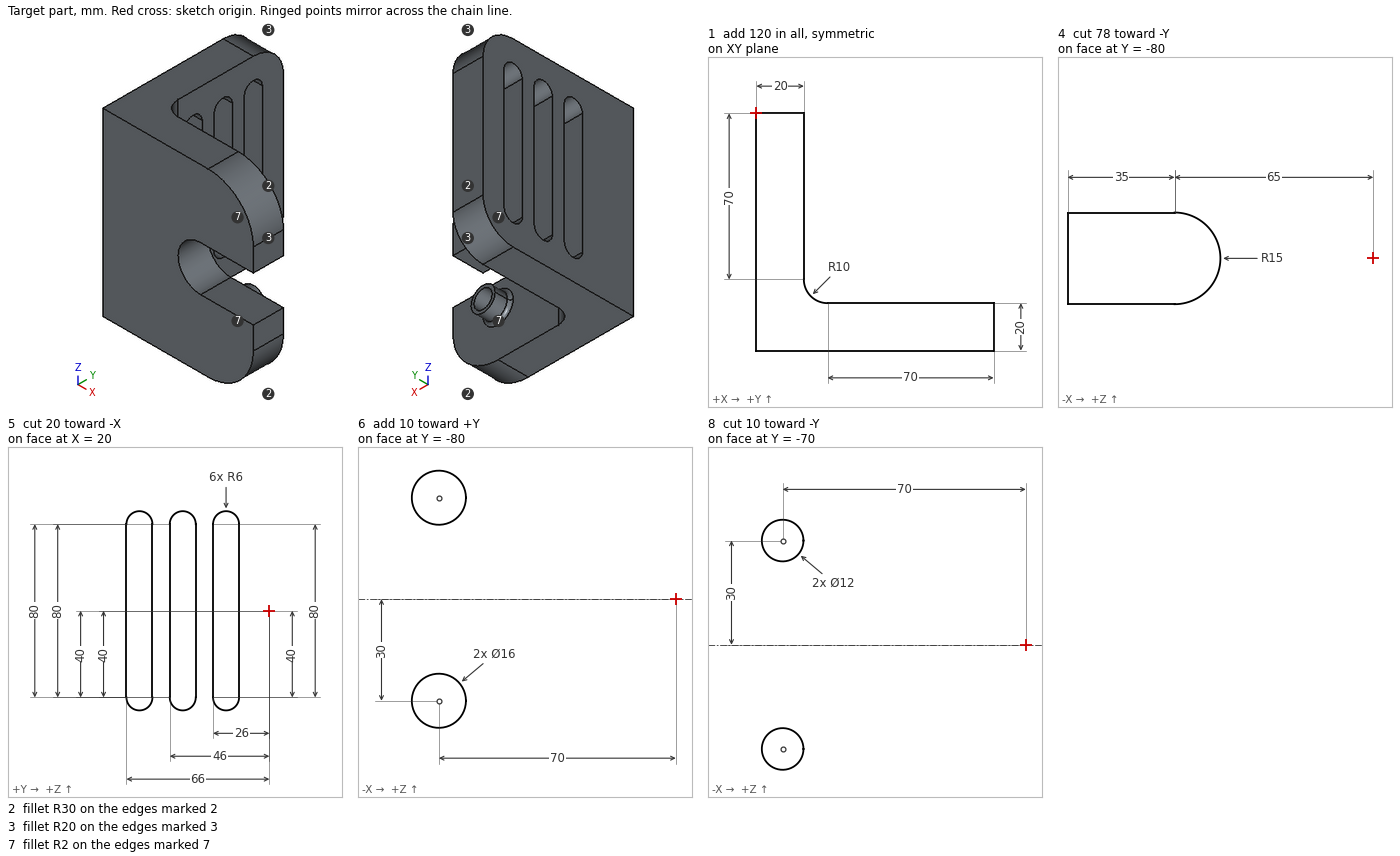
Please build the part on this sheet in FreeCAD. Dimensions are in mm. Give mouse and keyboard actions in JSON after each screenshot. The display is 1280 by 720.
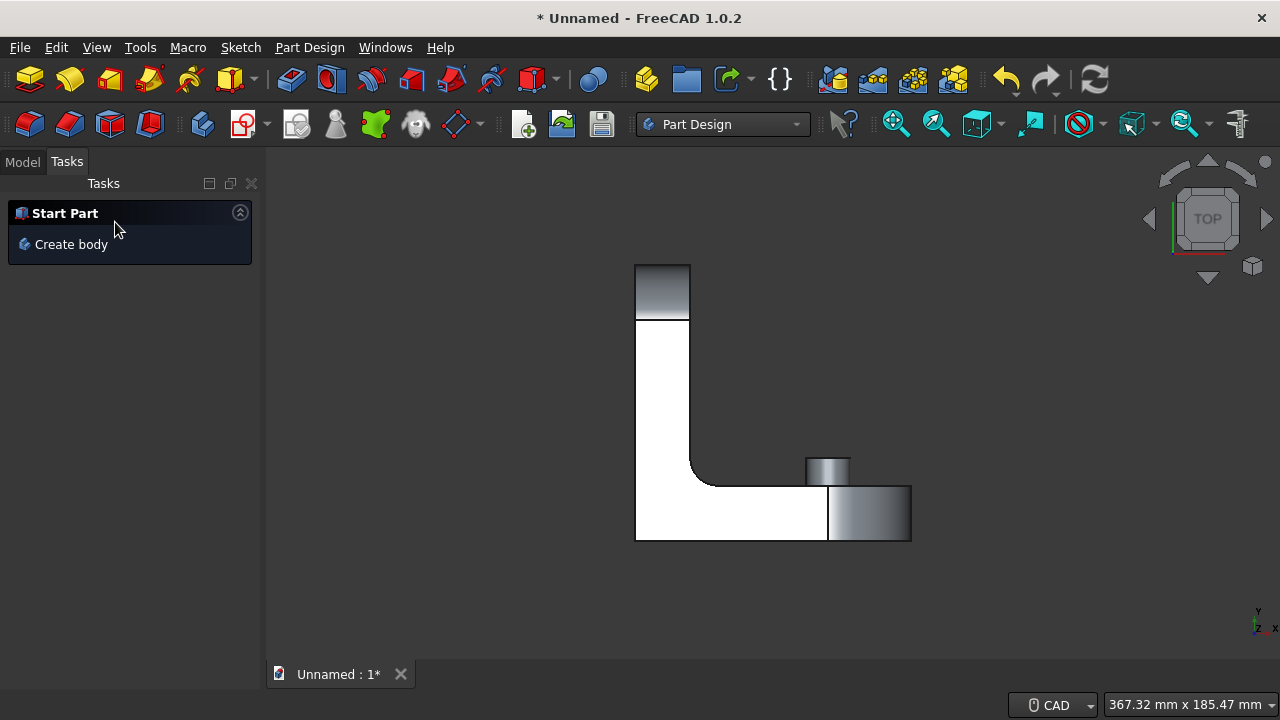
{"action": "key", "text": "1"}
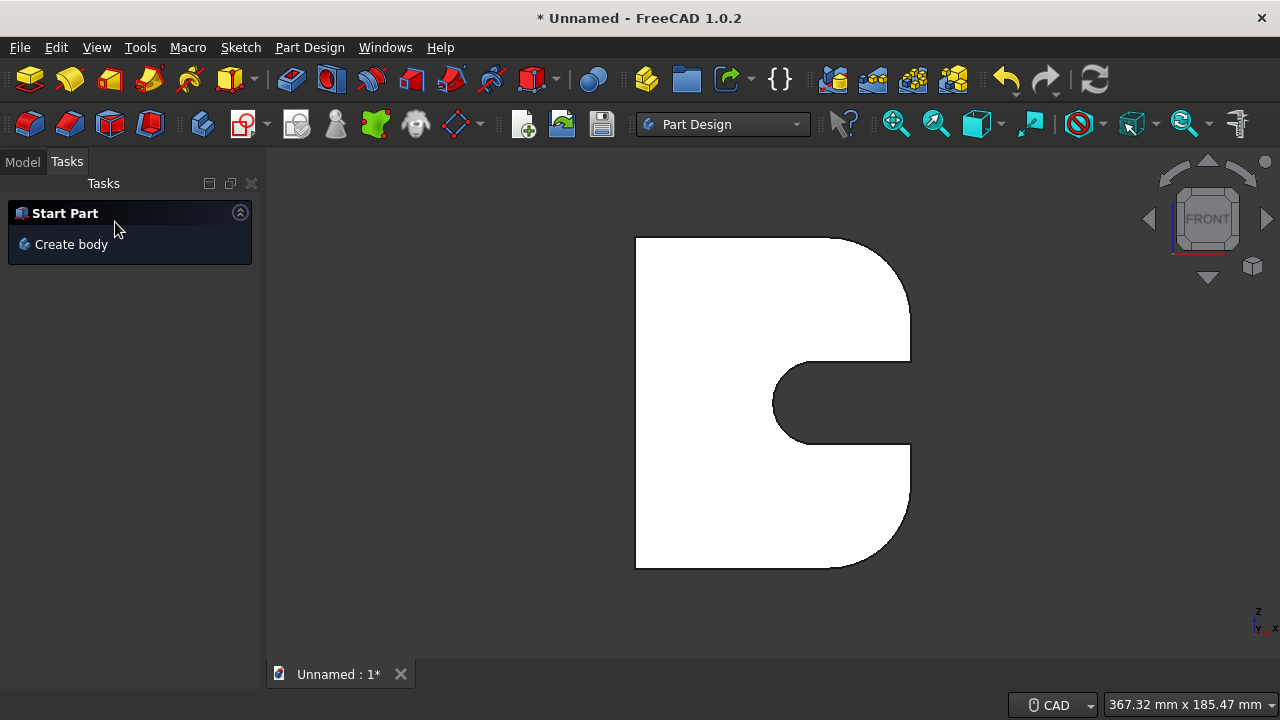
{"action": "key", "text": "3"}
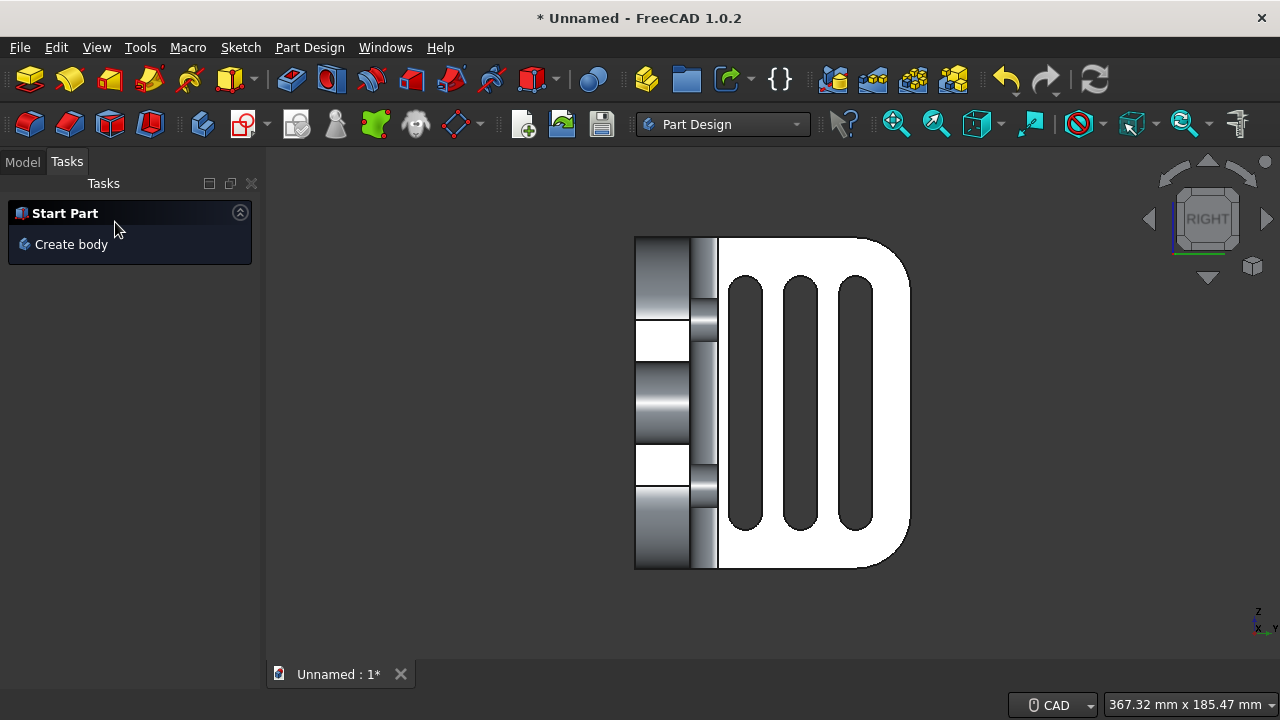
{"action": "key", "text": "5"}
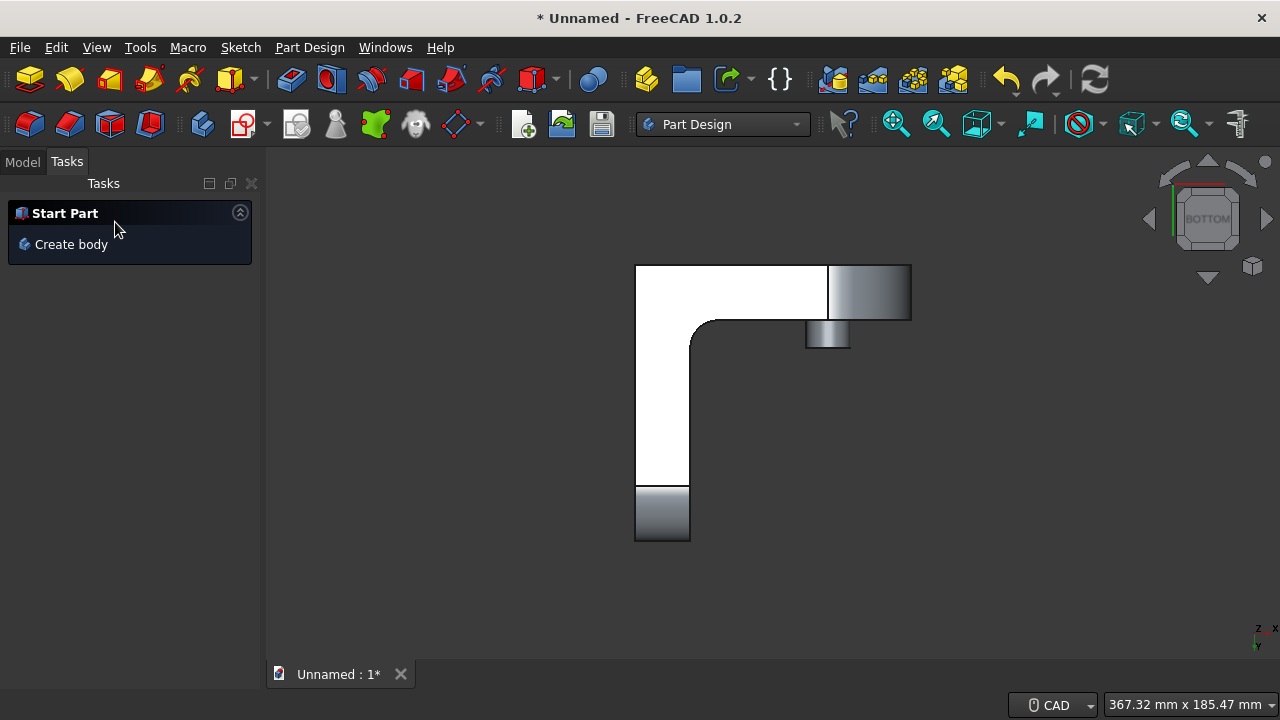
{"action": "key", "text": "4"}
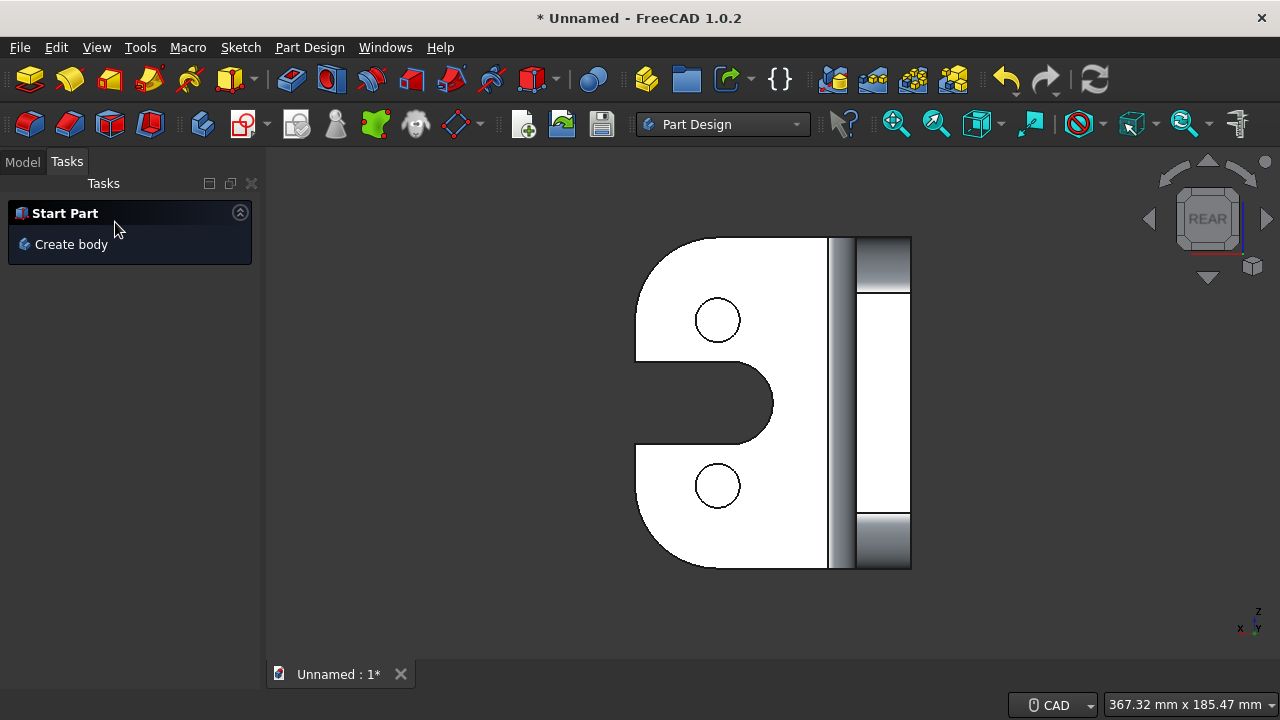
{"action": "key", "text": "6"}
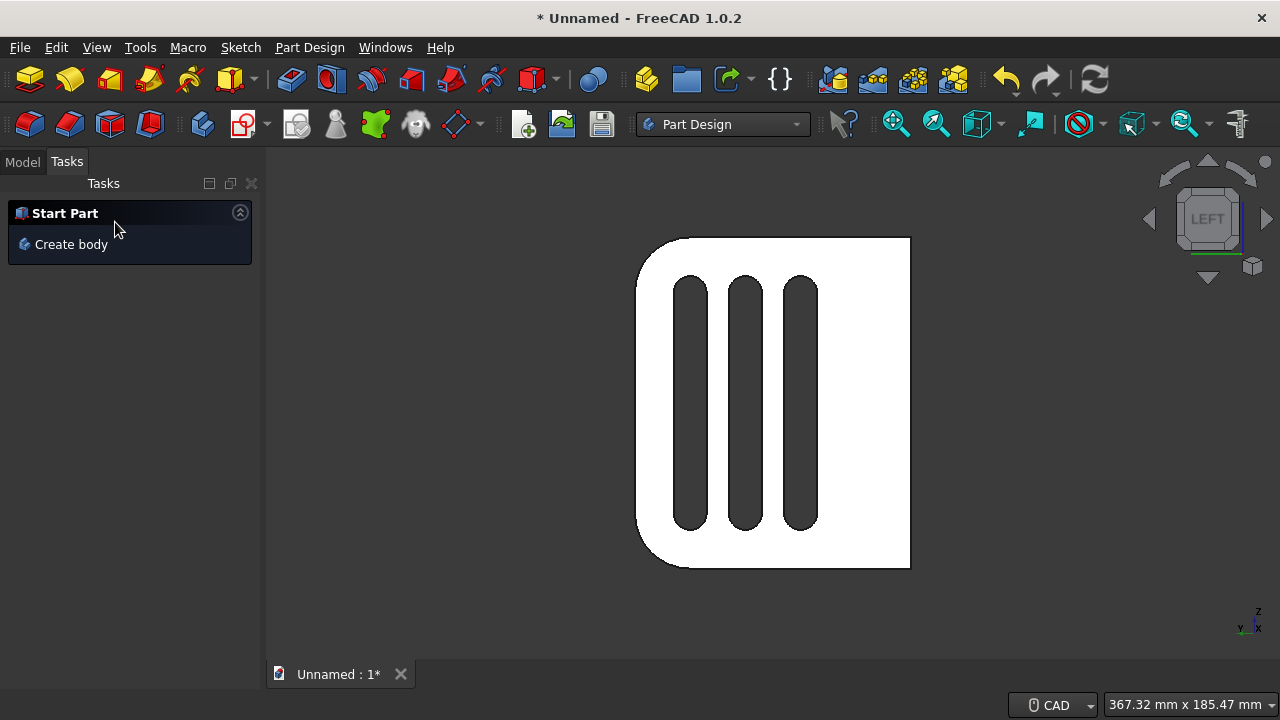
{"action": "key", "text": "v 3"}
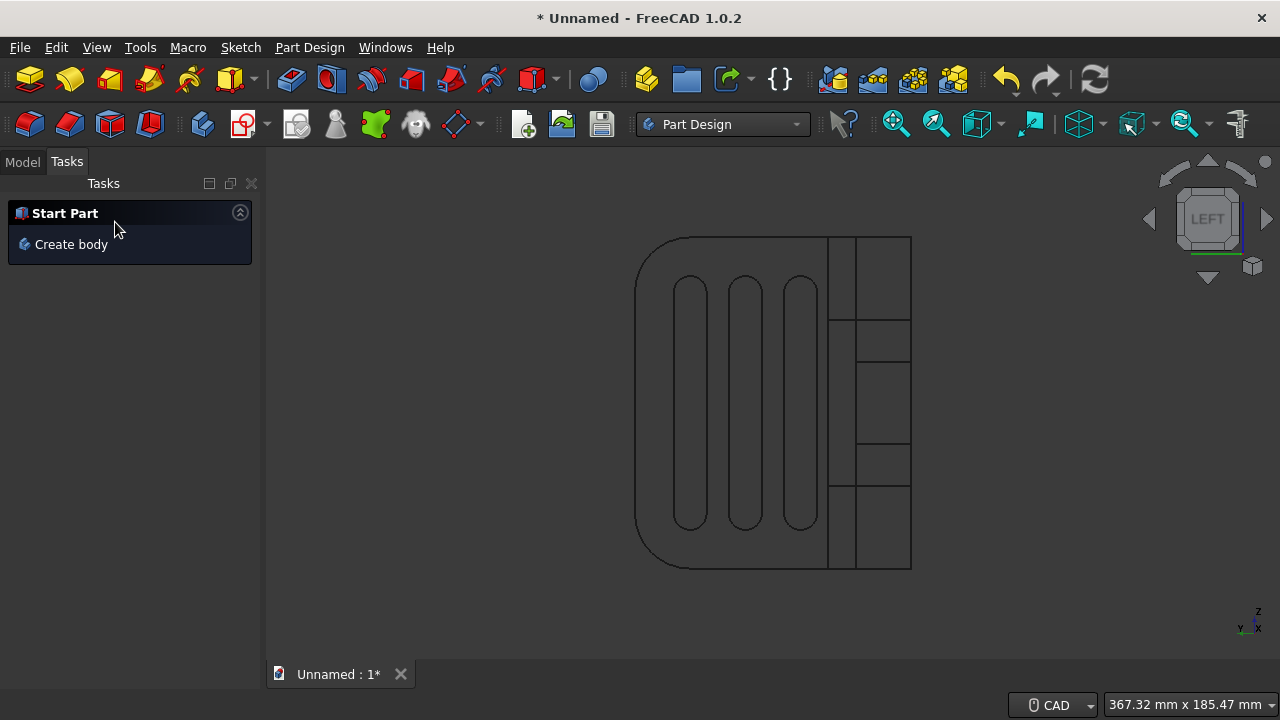
{"action": "key", "text": "0"}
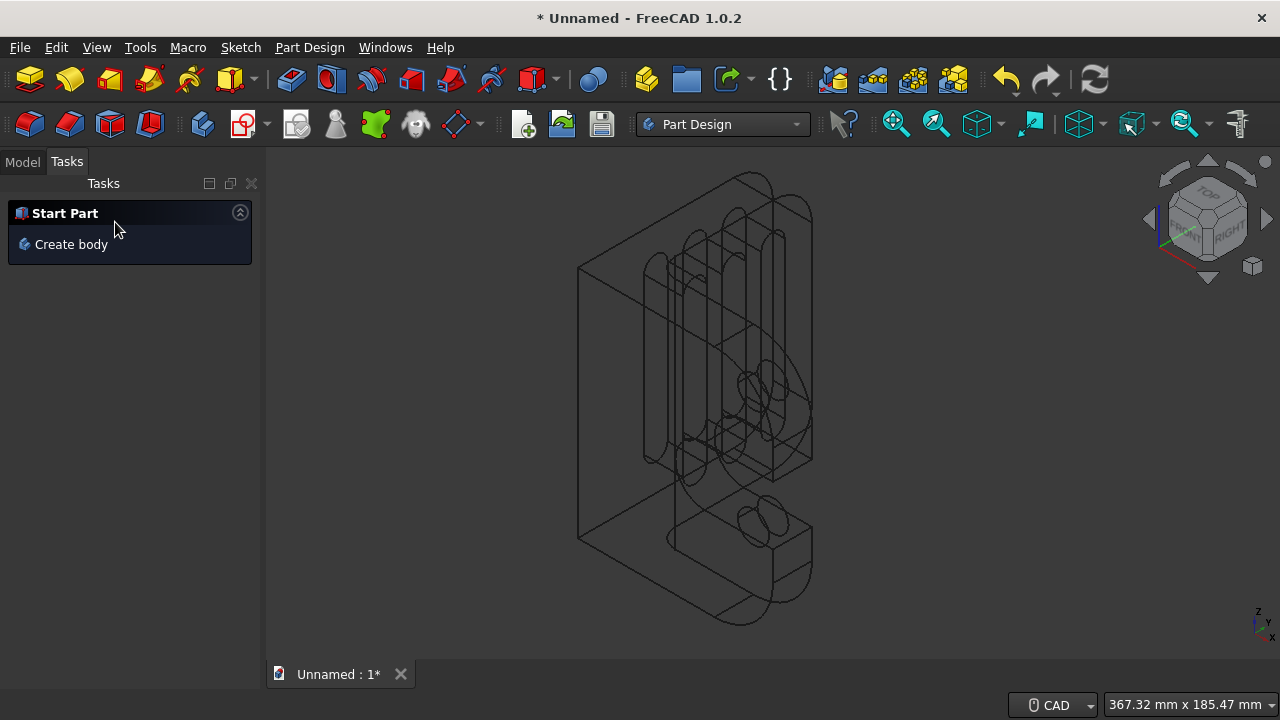
{"action": "left_click", "coordinate": [769, 535]}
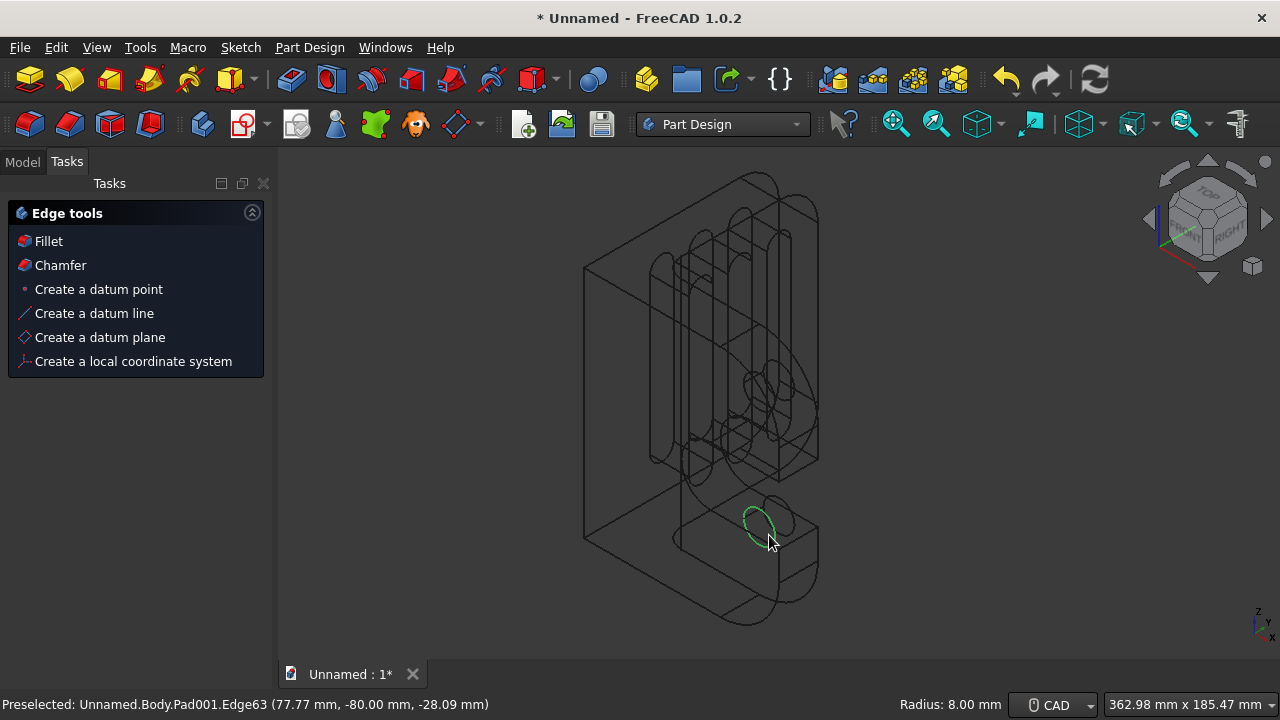
{"action": "left_click", "coordinate": [775, 400], "text": "ctrl"}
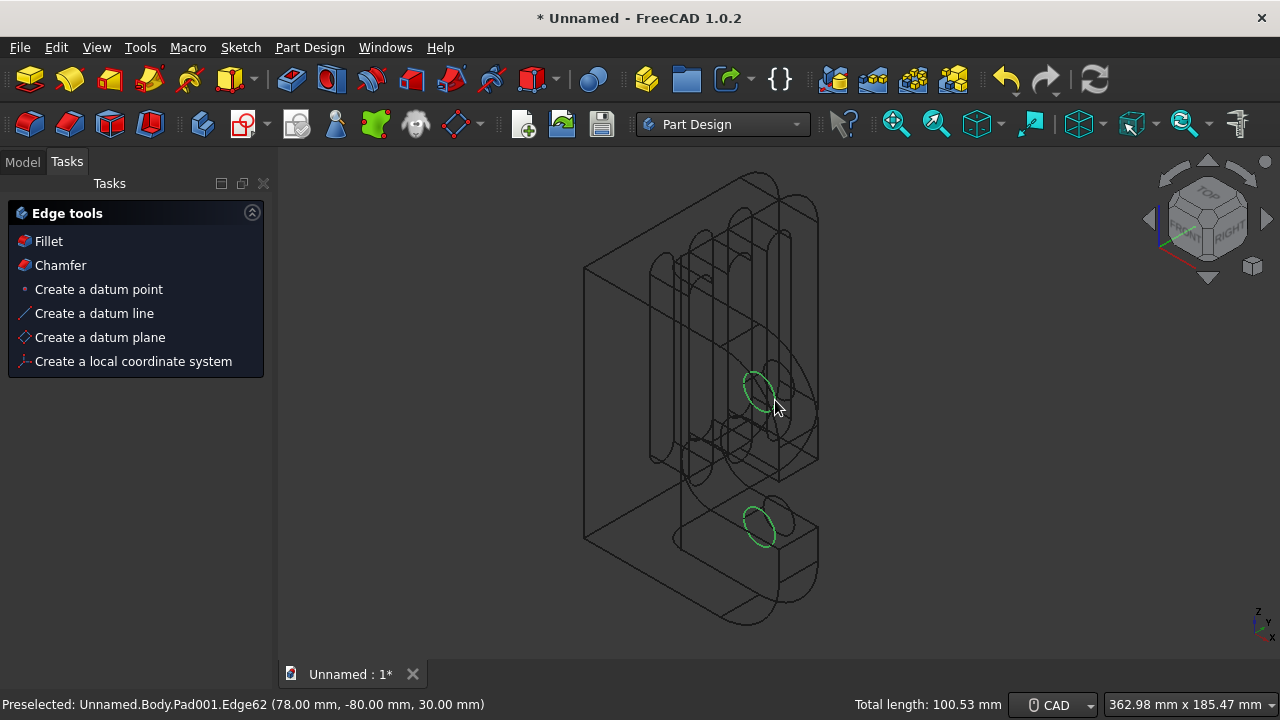
{"action": "key", "text": "v 1"}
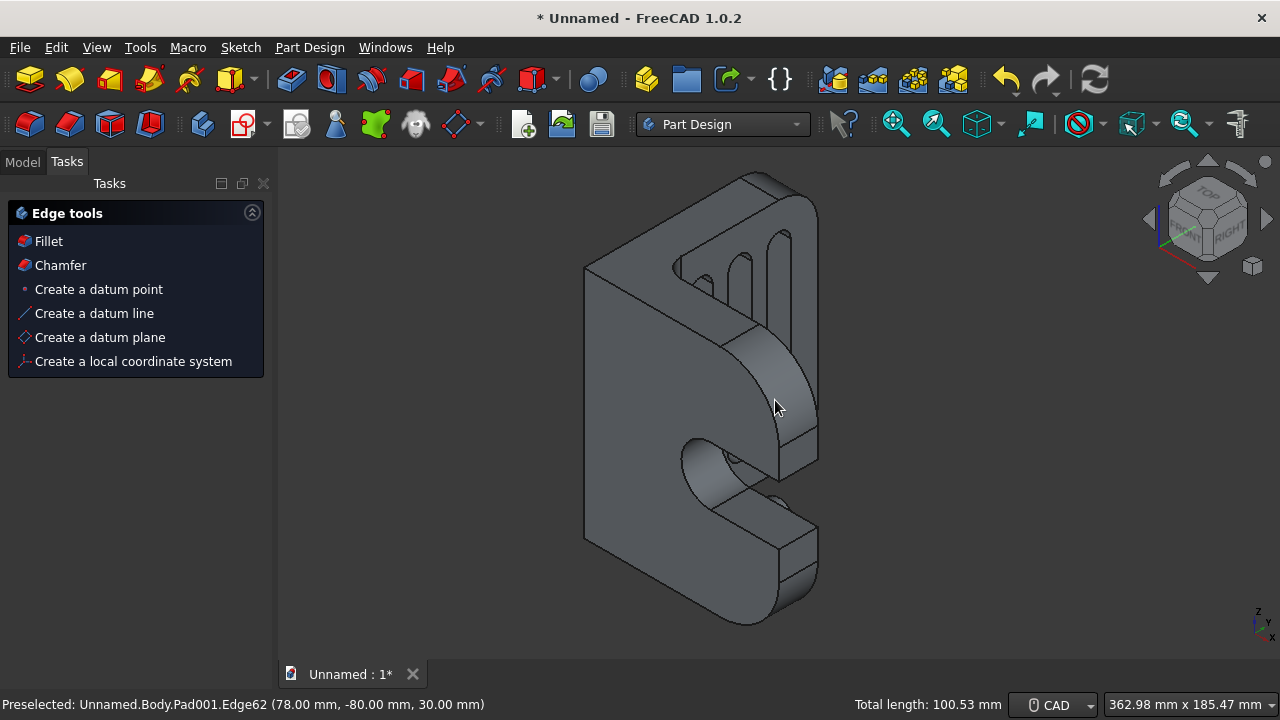
{"action": "left_click", "coordinate": [30, 124]}